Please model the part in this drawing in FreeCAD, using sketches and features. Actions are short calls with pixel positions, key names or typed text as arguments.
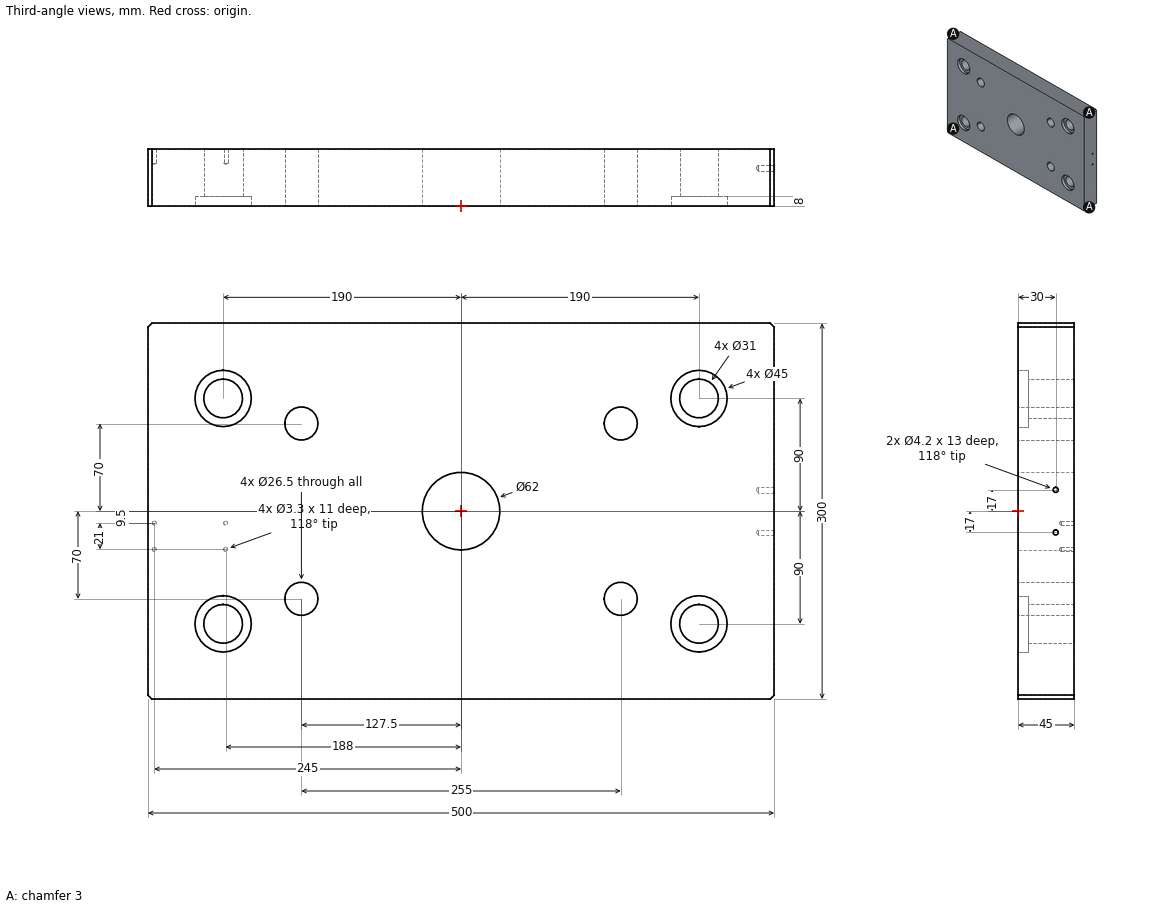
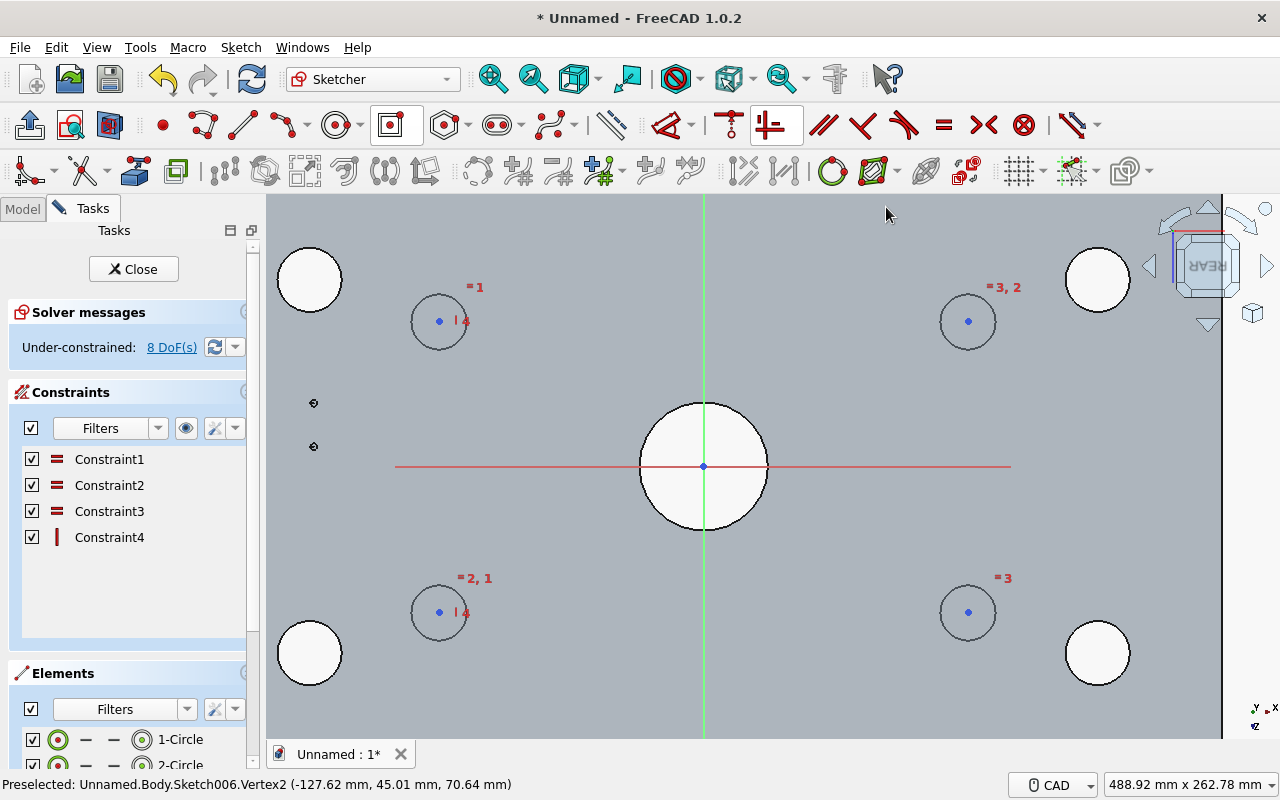
click(439, 322)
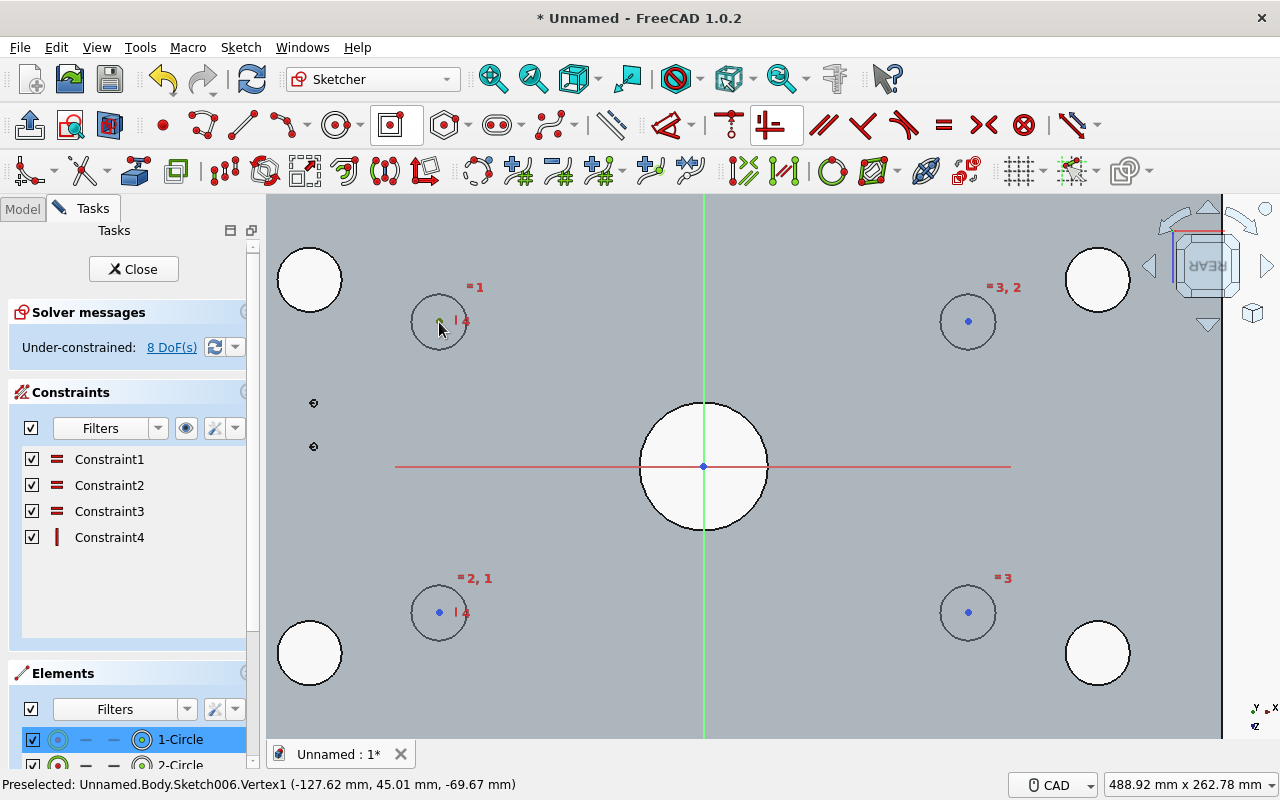
click(968, 322)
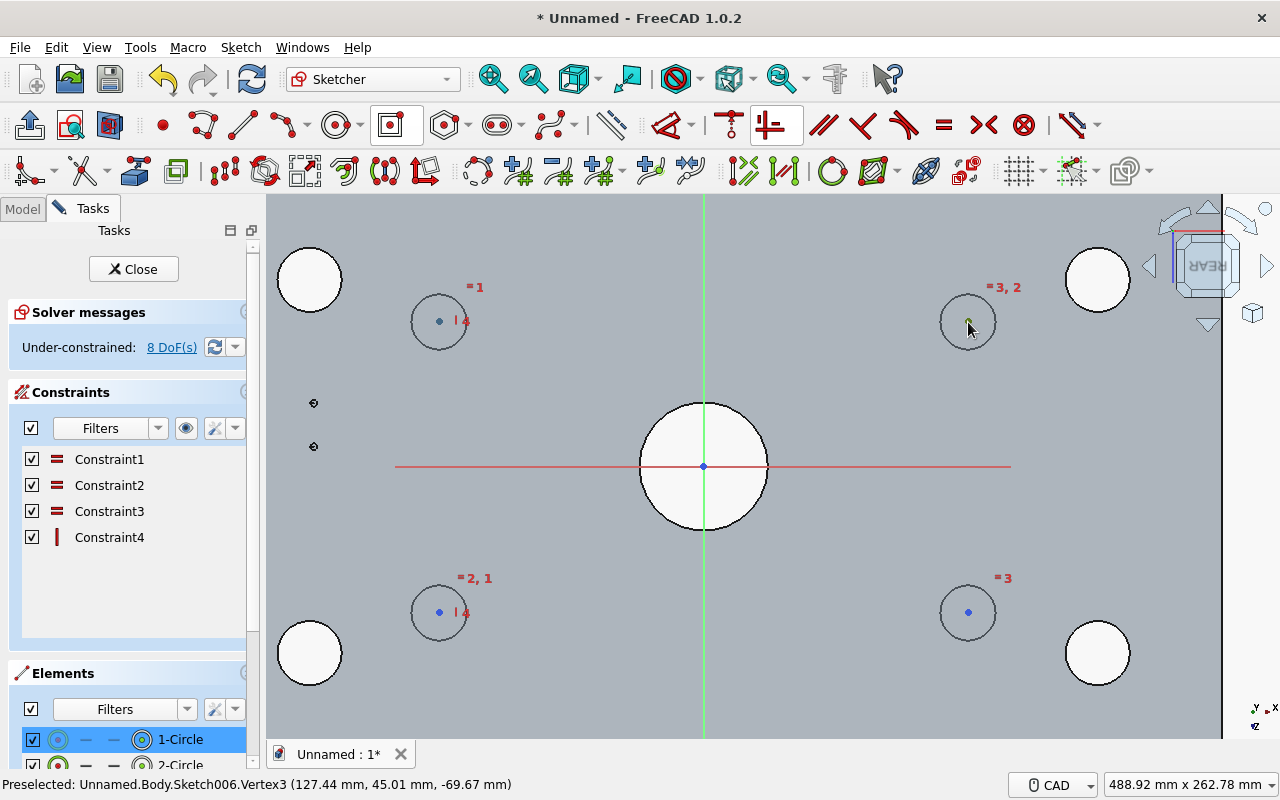
key(h)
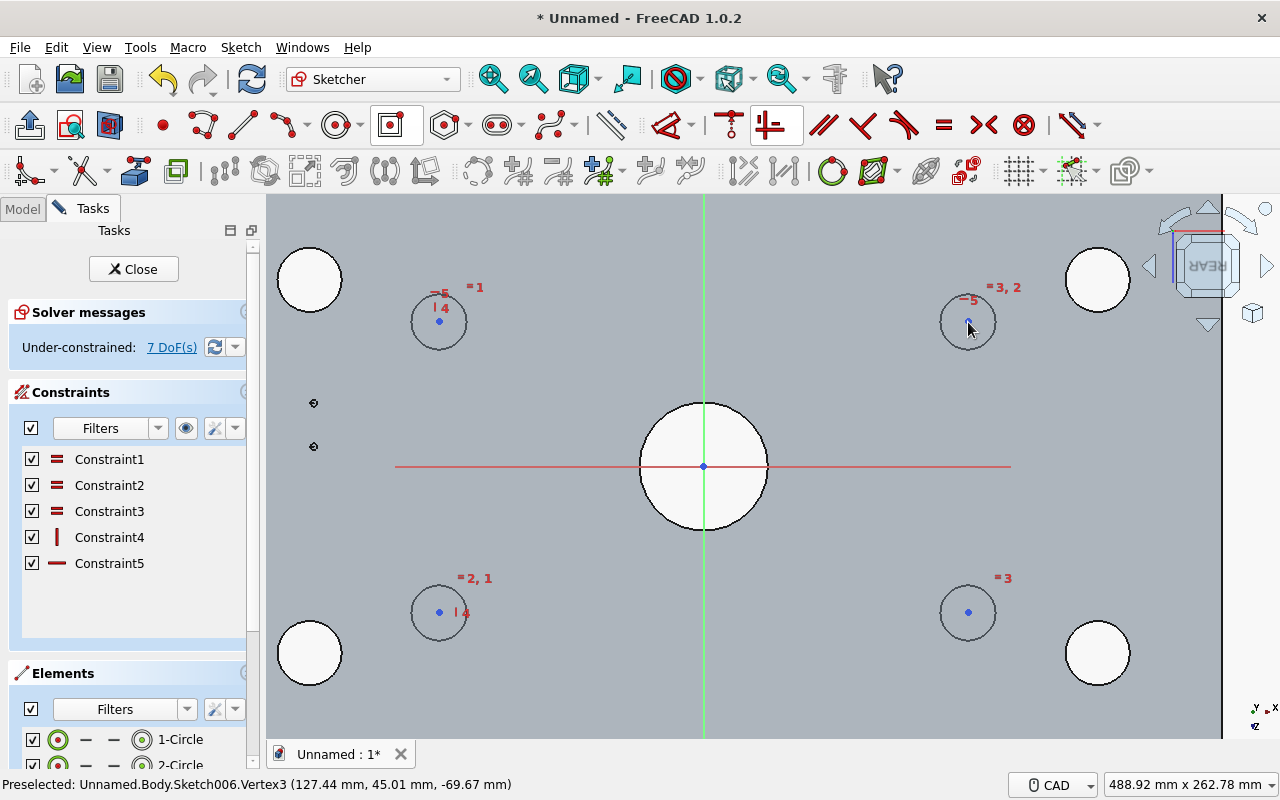
click(968, 322)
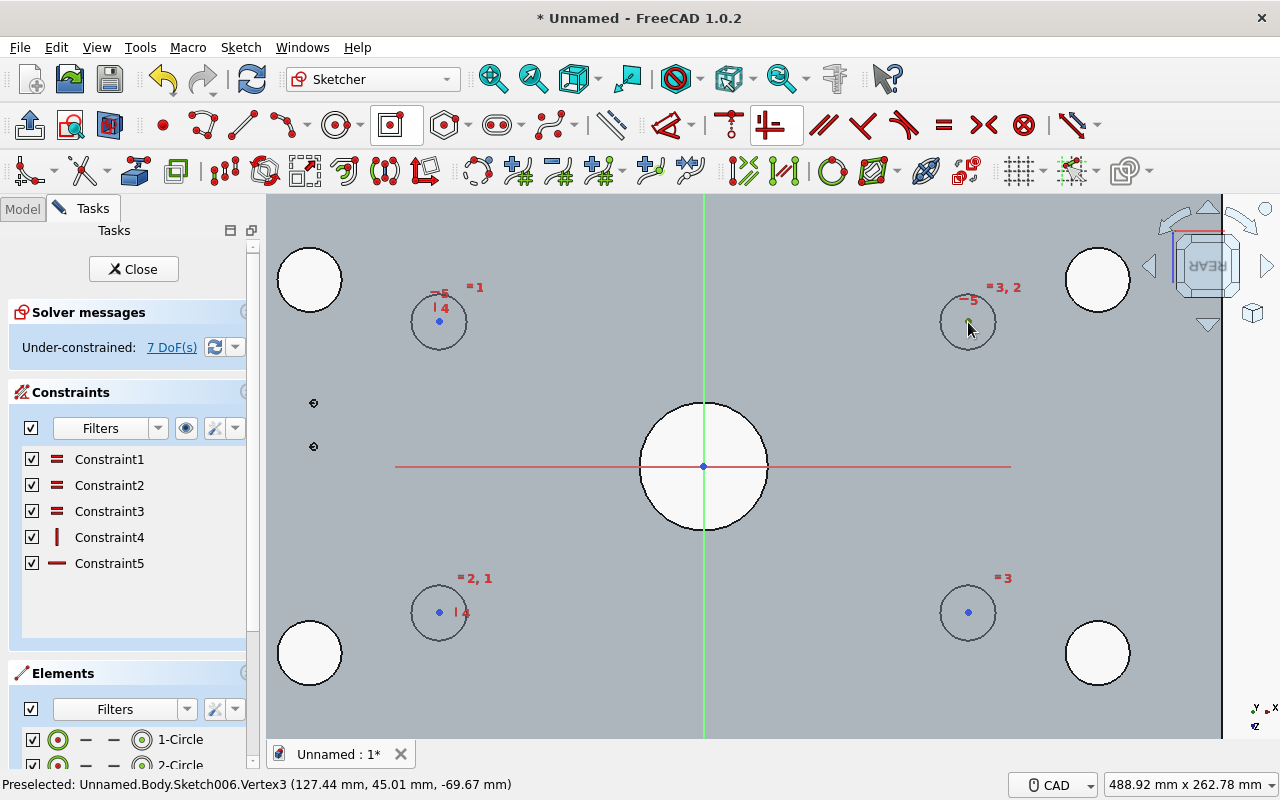
click(968, 613)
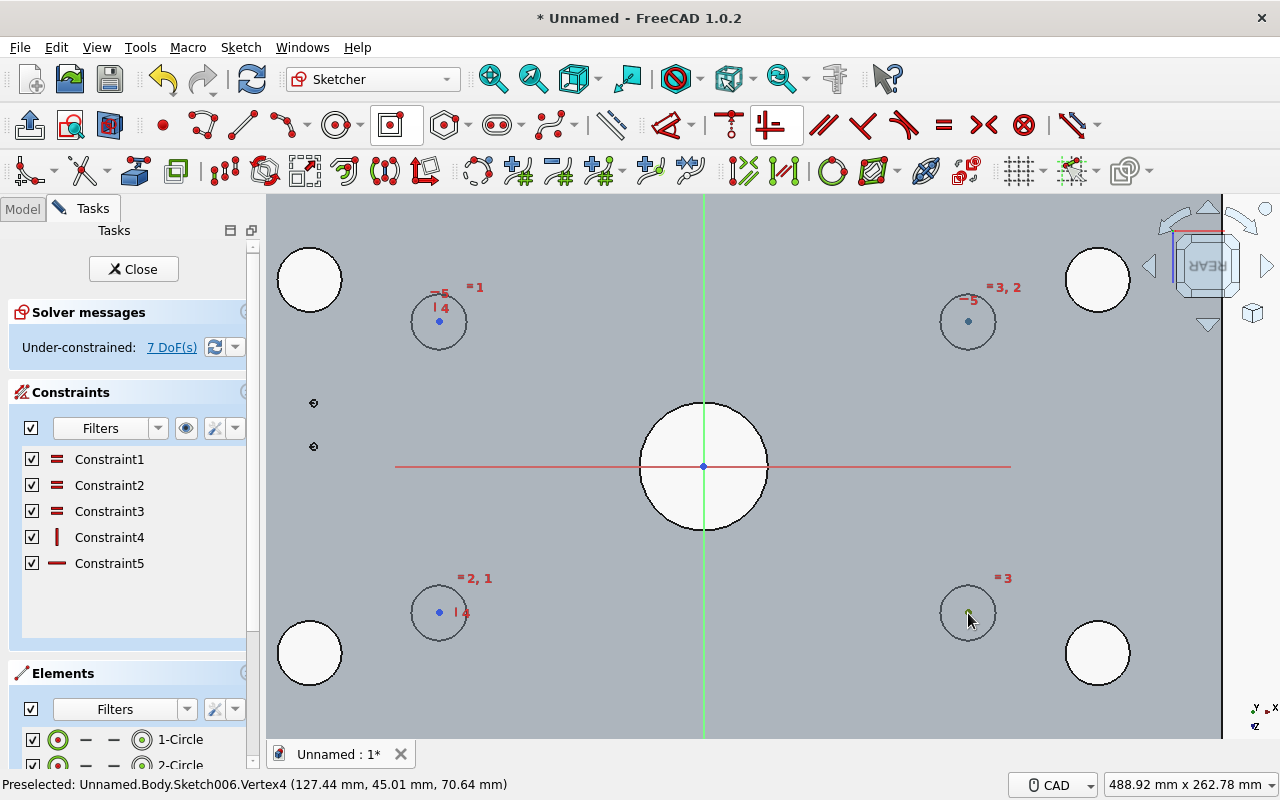
key(v)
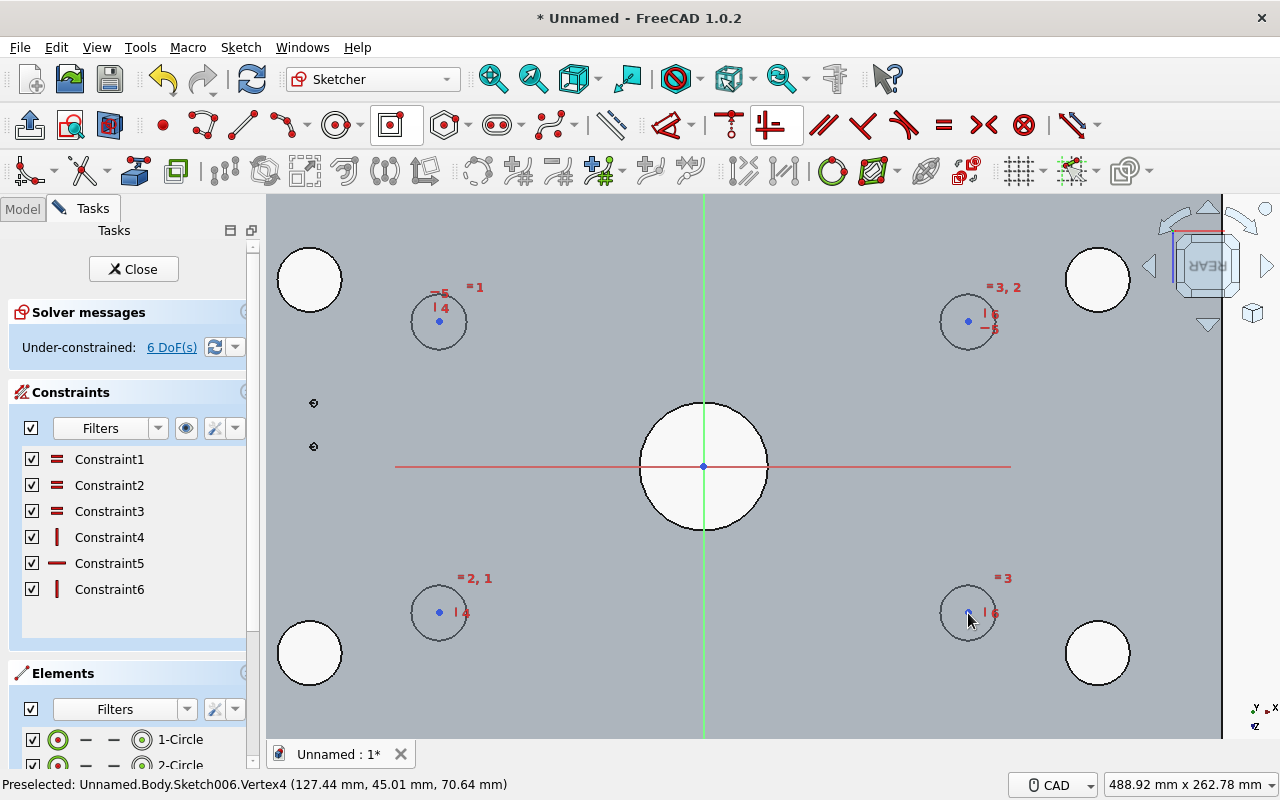
click(439, 613)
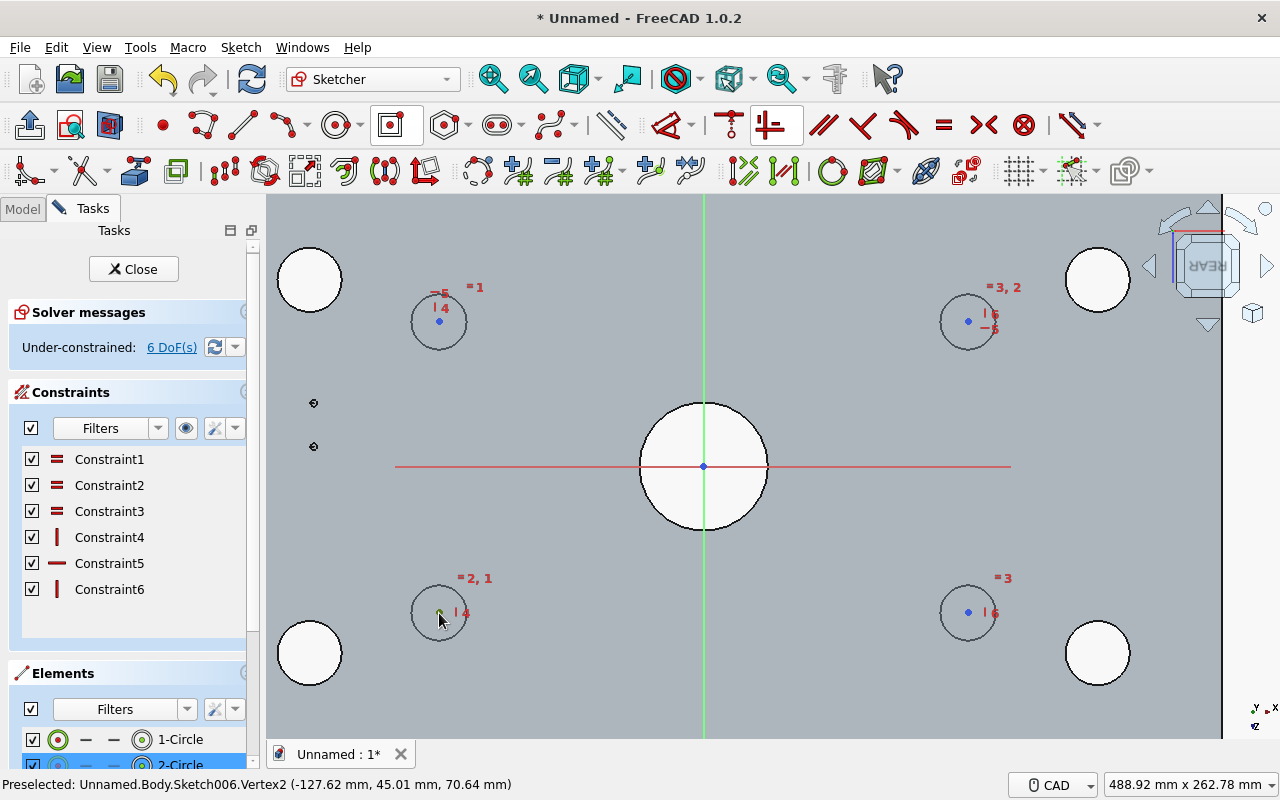
click(968, 613)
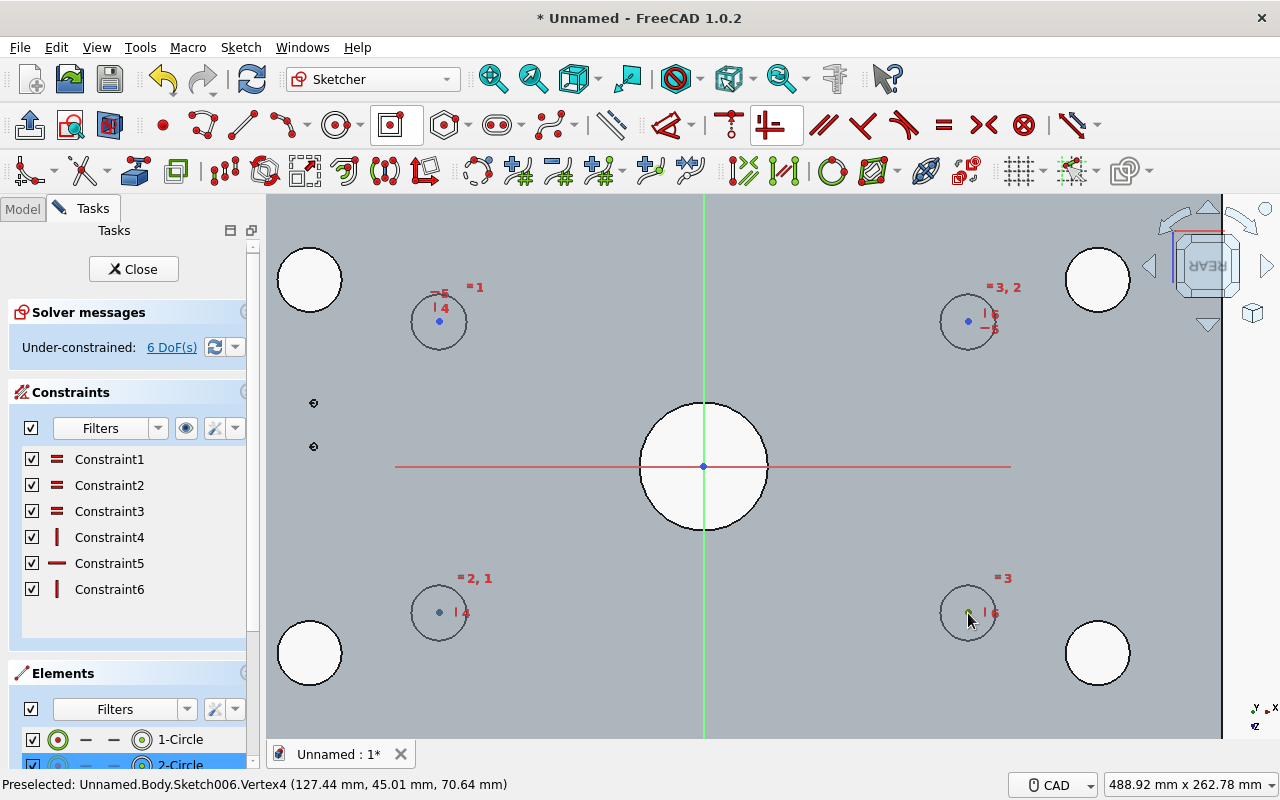
click(798, 126)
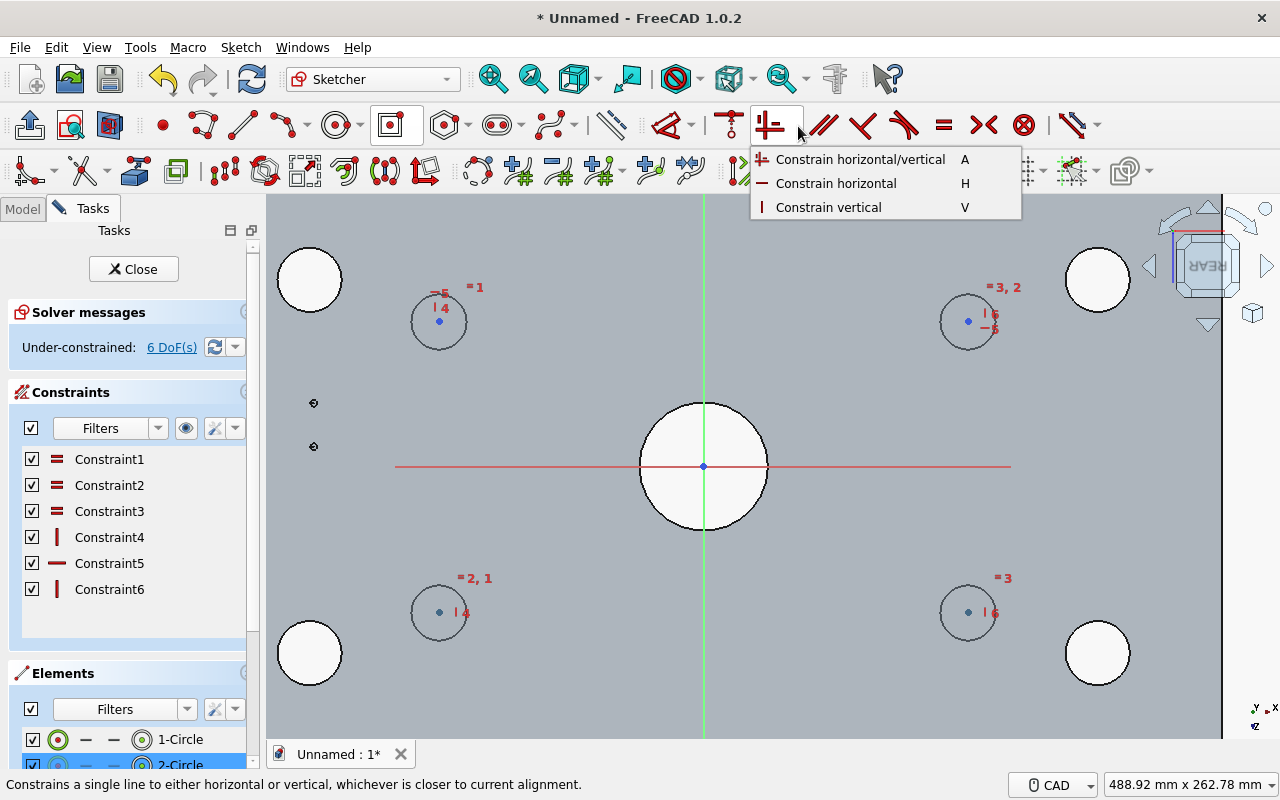
click(886, 183)